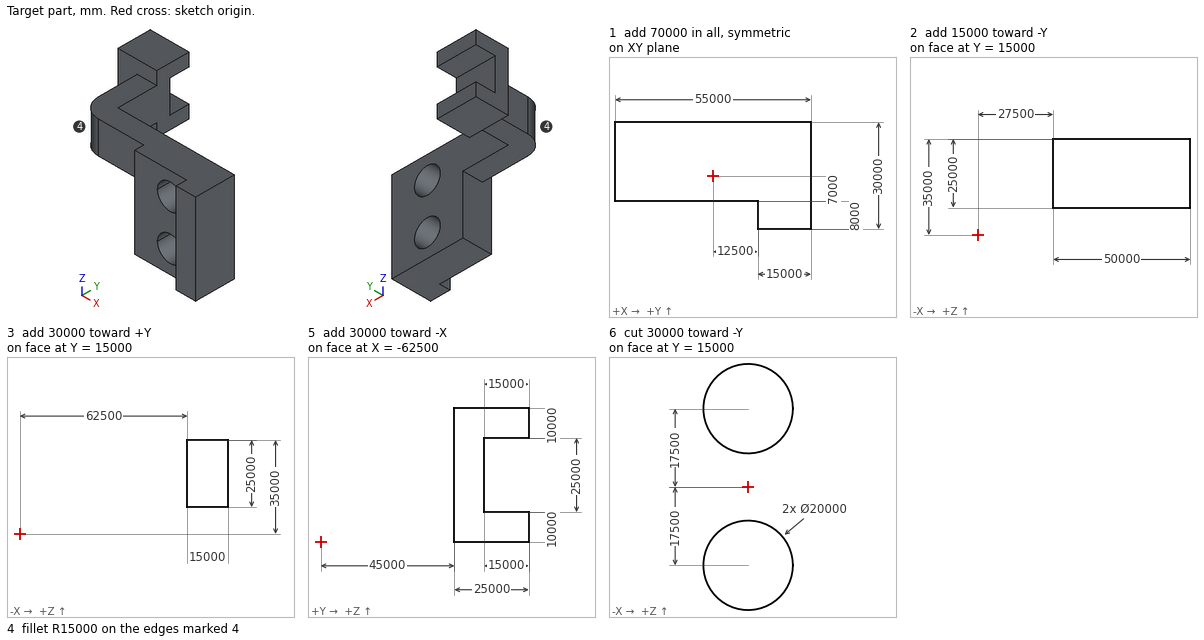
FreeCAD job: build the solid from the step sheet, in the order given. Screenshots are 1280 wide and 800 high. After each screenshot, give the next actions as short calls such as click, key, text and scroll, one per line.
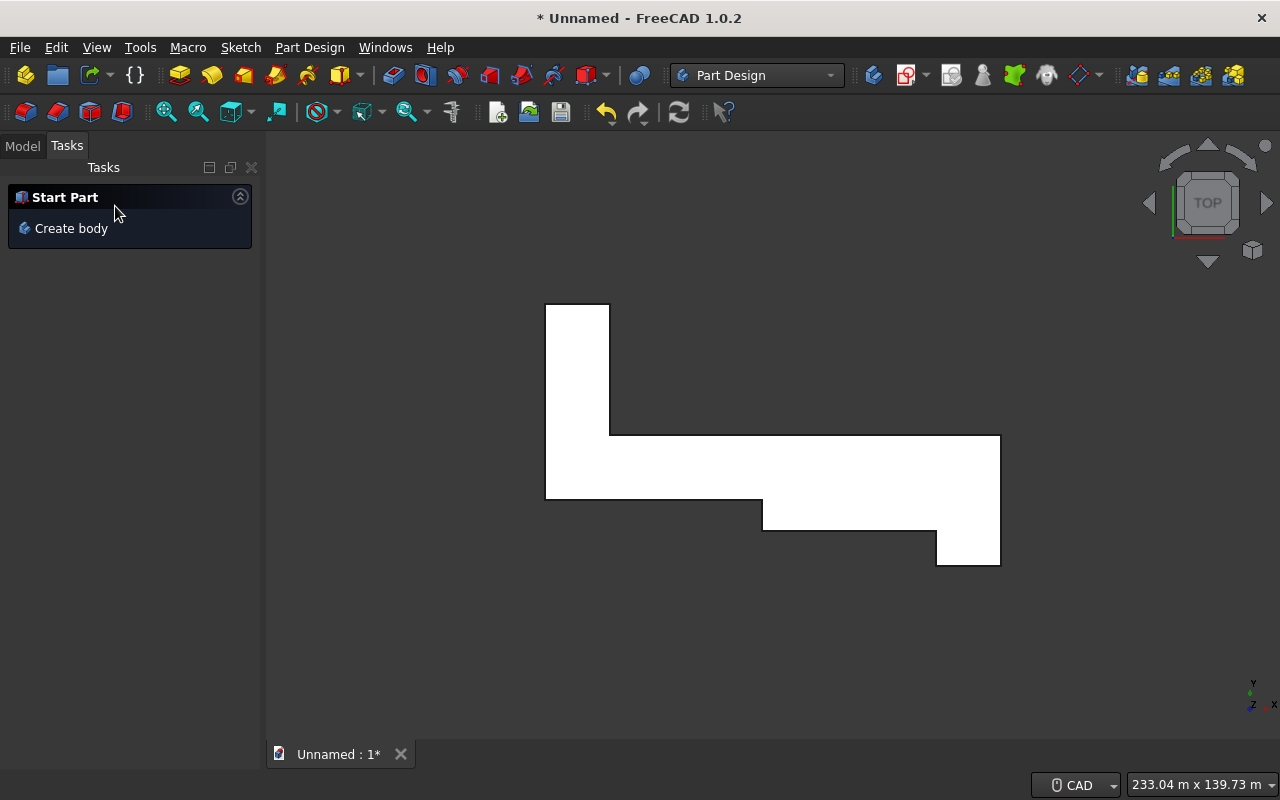
key(v)
key(f)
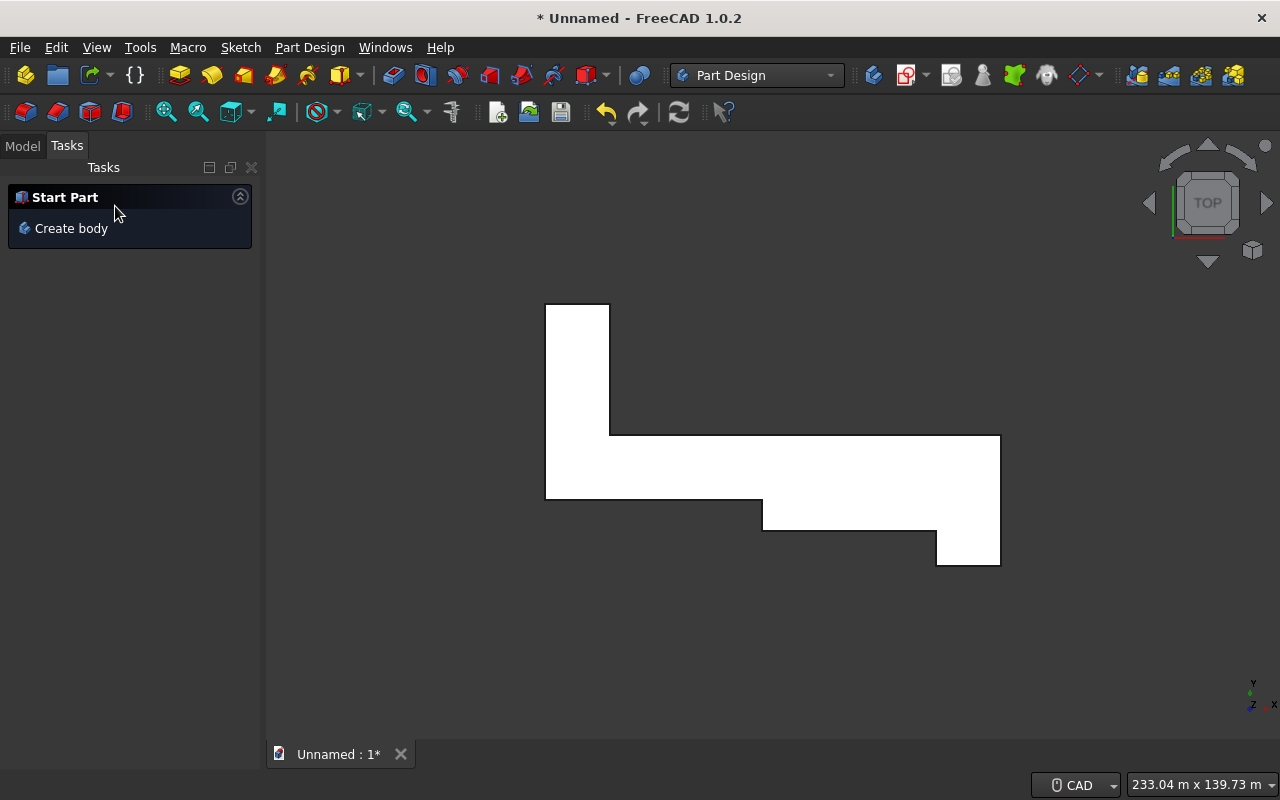
key(1)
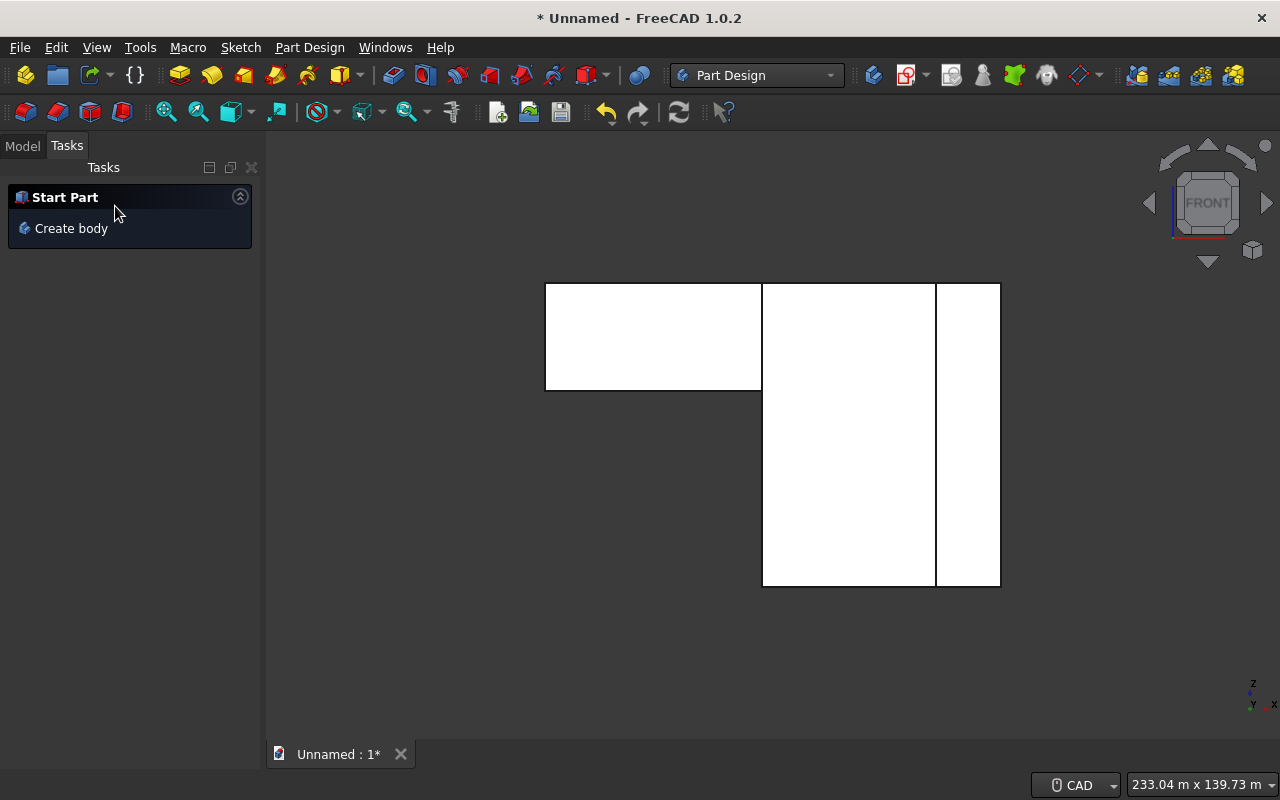
click(545, 336)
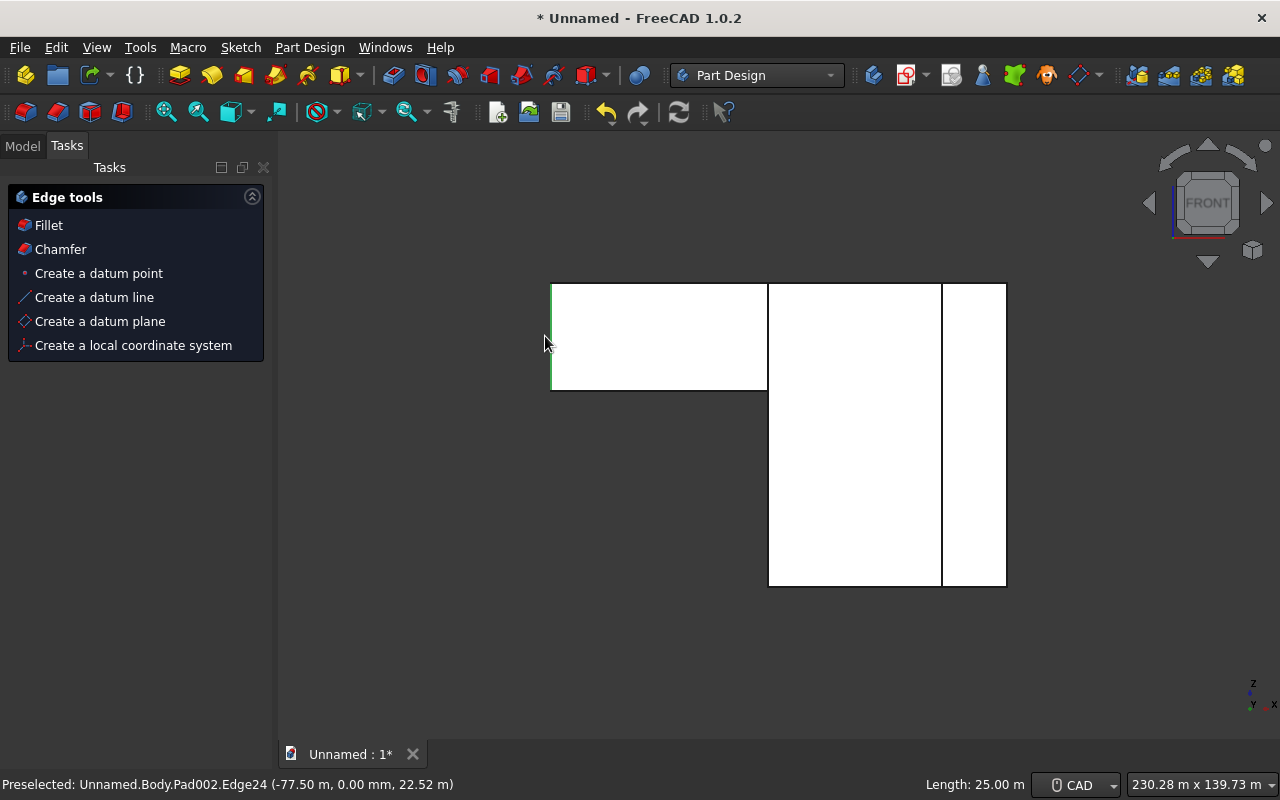
click(26, 112)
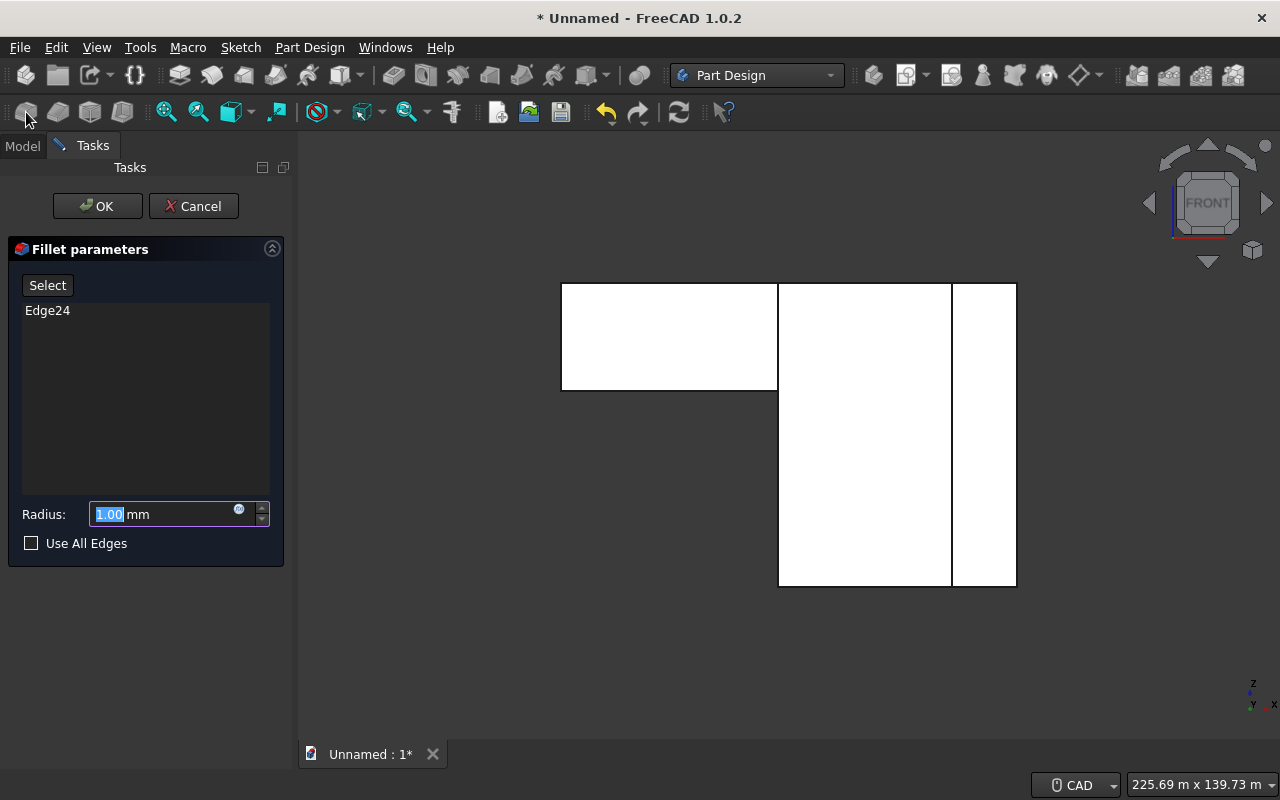
text(15000)
key(Tab)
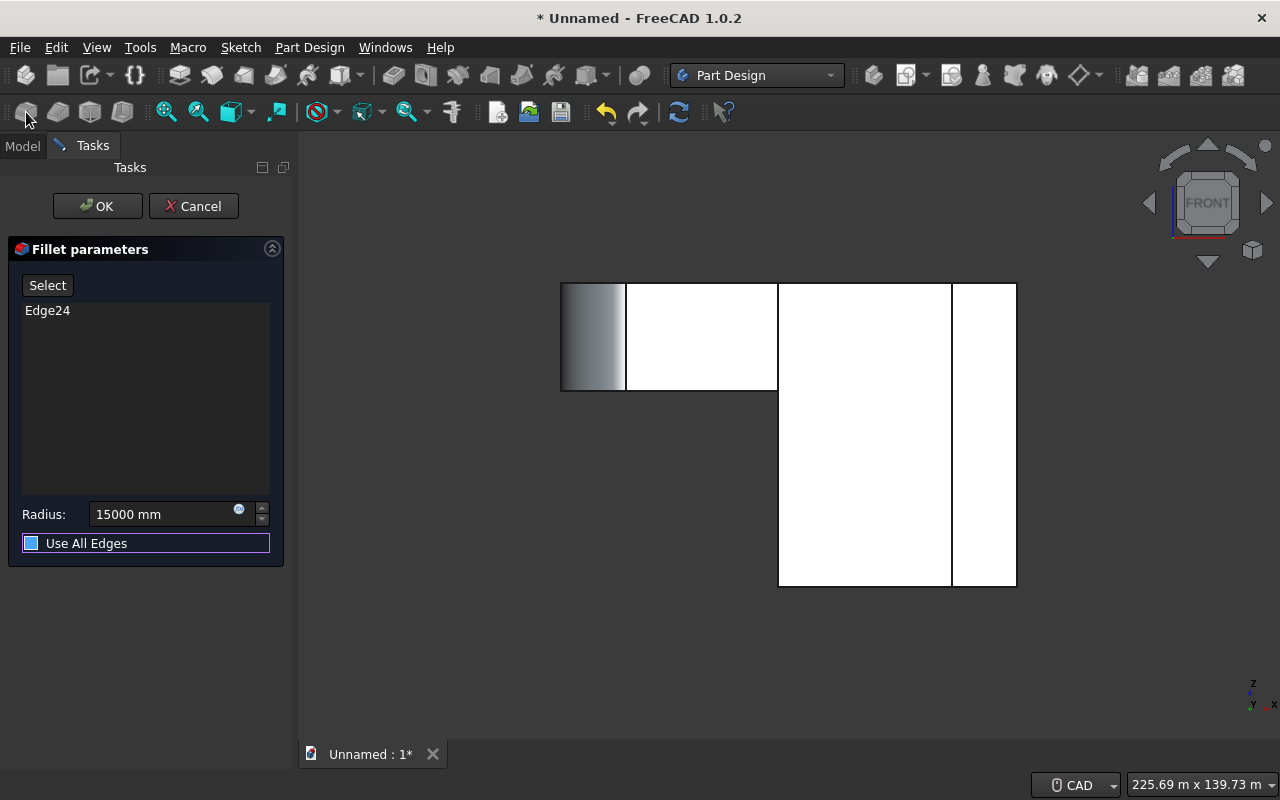
click(98, 206)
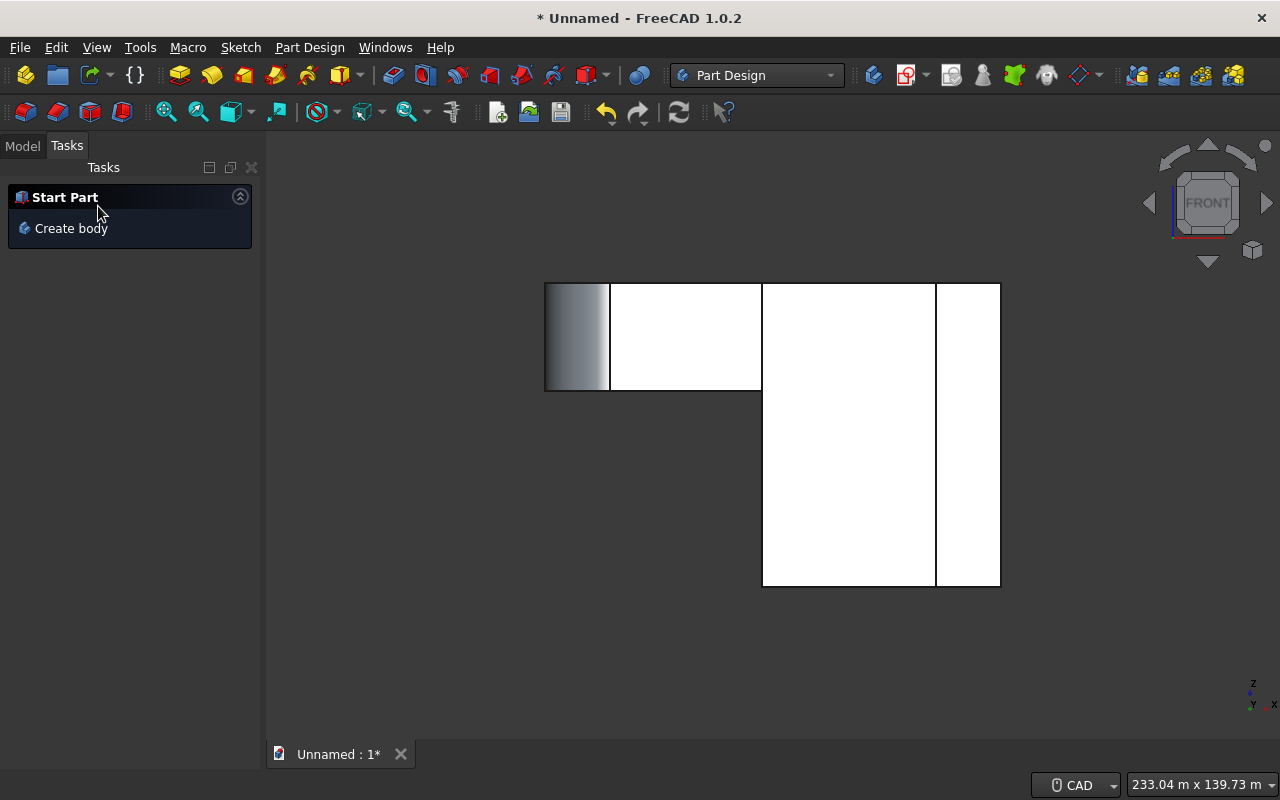
key(0)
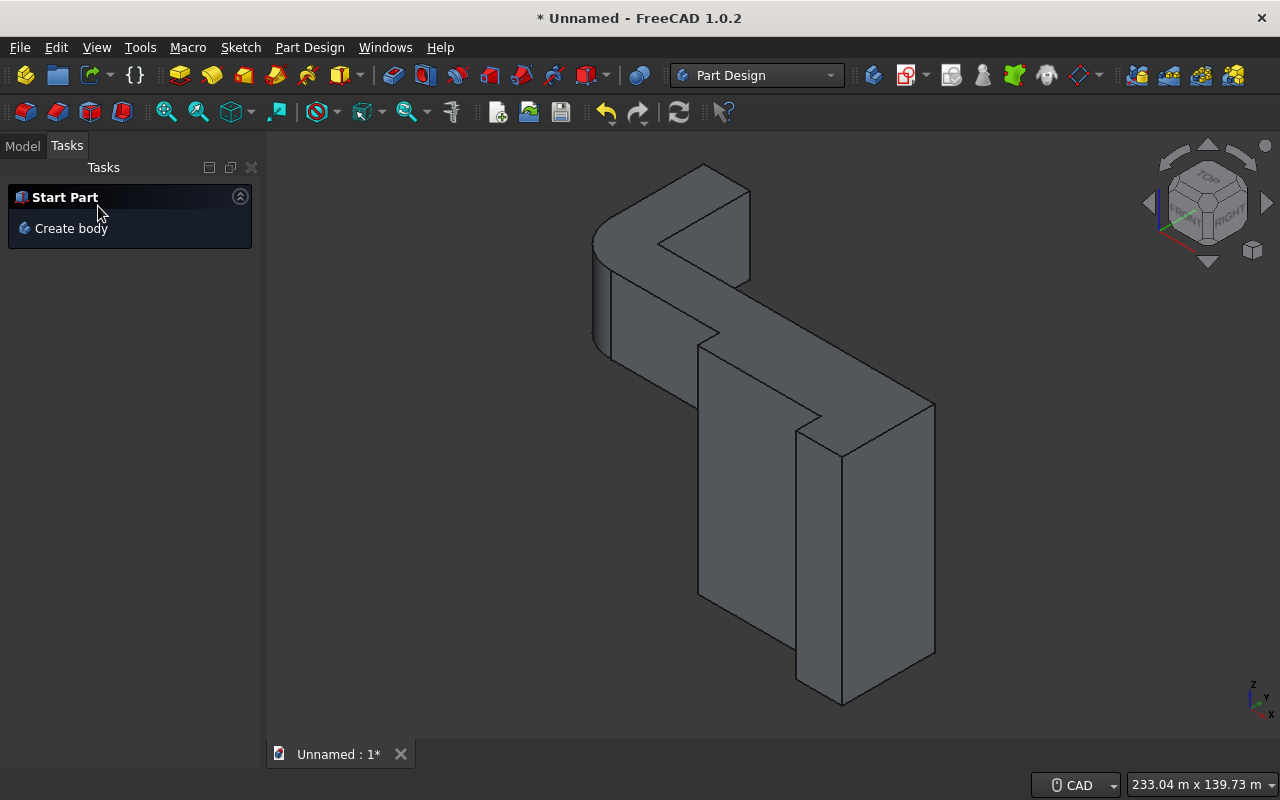
click(717, 253)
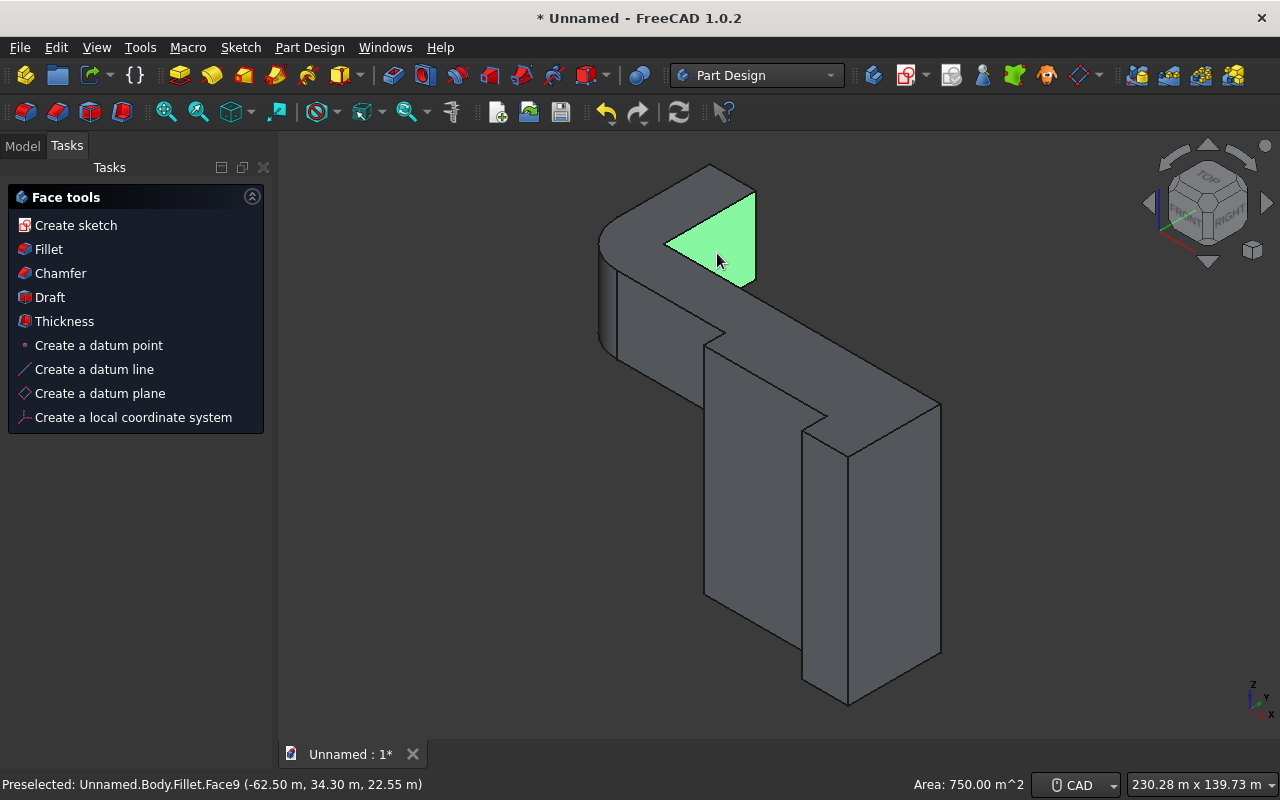
click(906, 76)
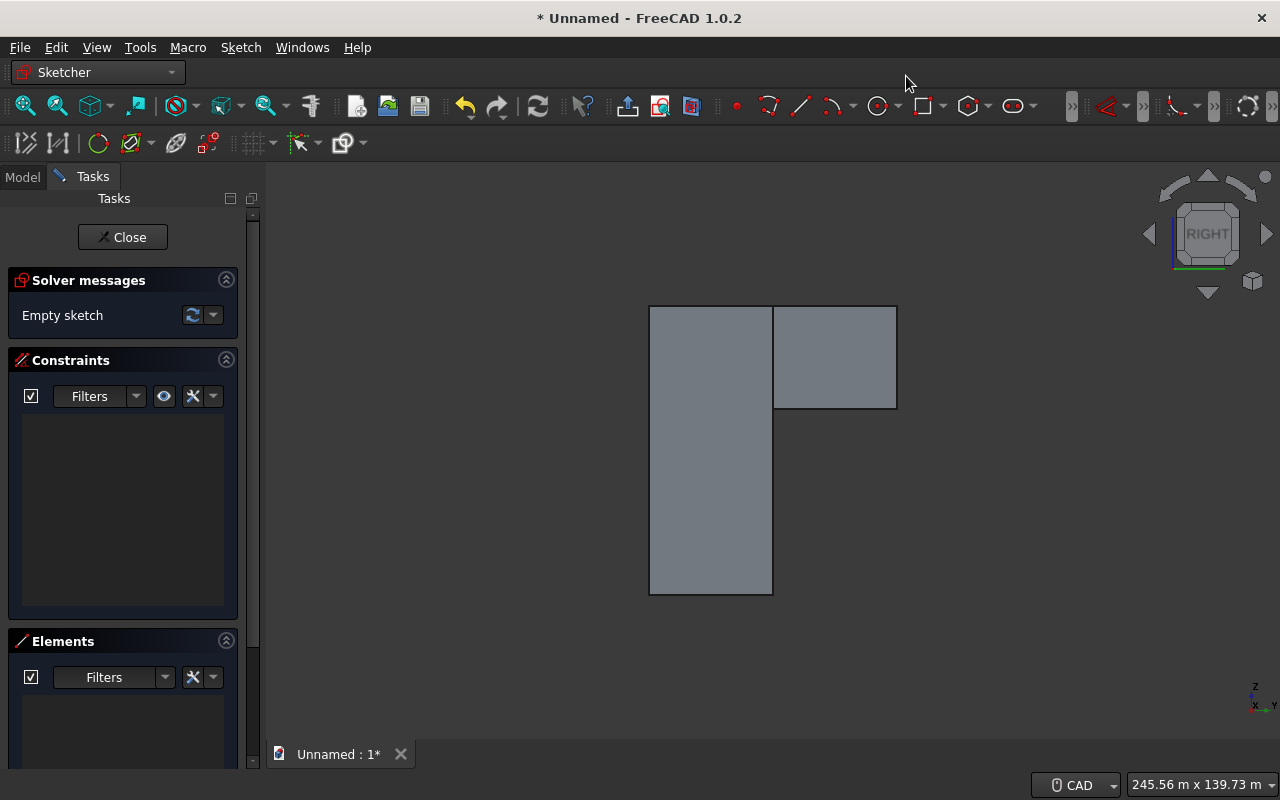
scroll(1039, 245, up, 3)